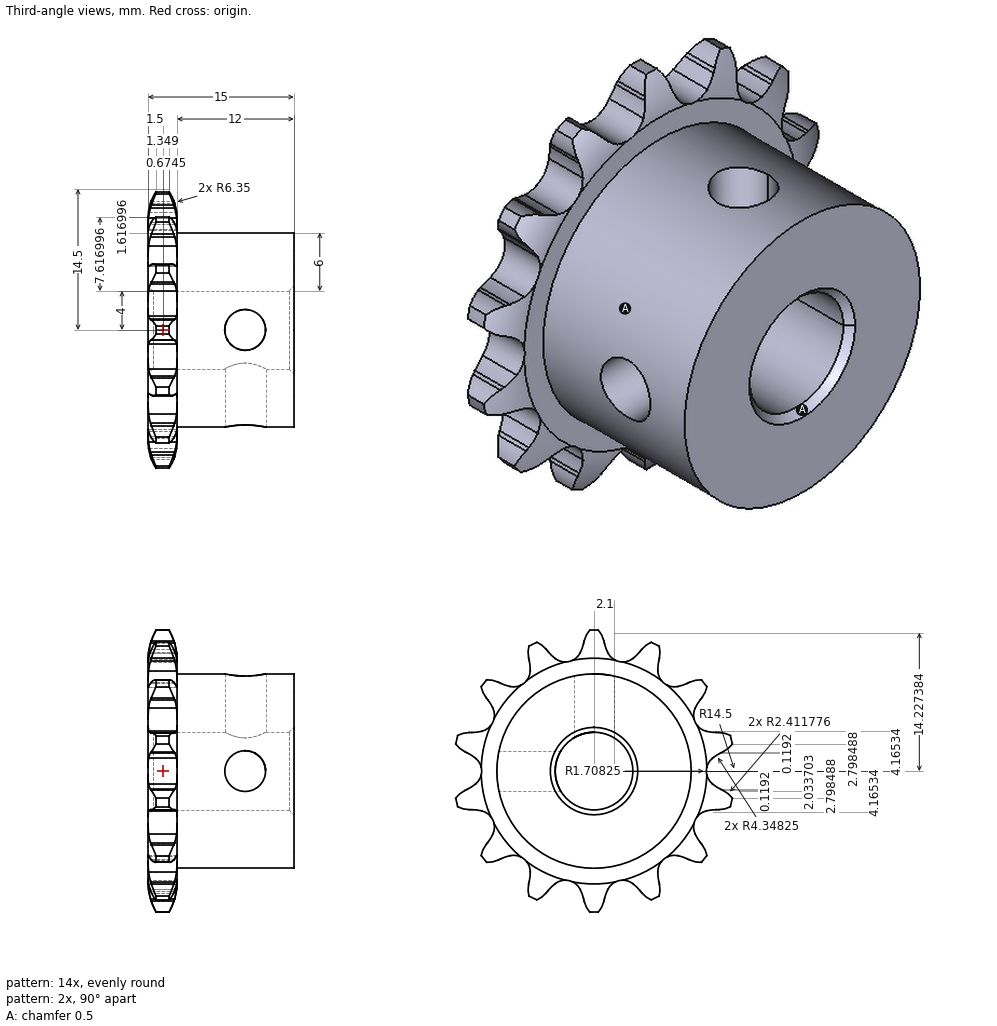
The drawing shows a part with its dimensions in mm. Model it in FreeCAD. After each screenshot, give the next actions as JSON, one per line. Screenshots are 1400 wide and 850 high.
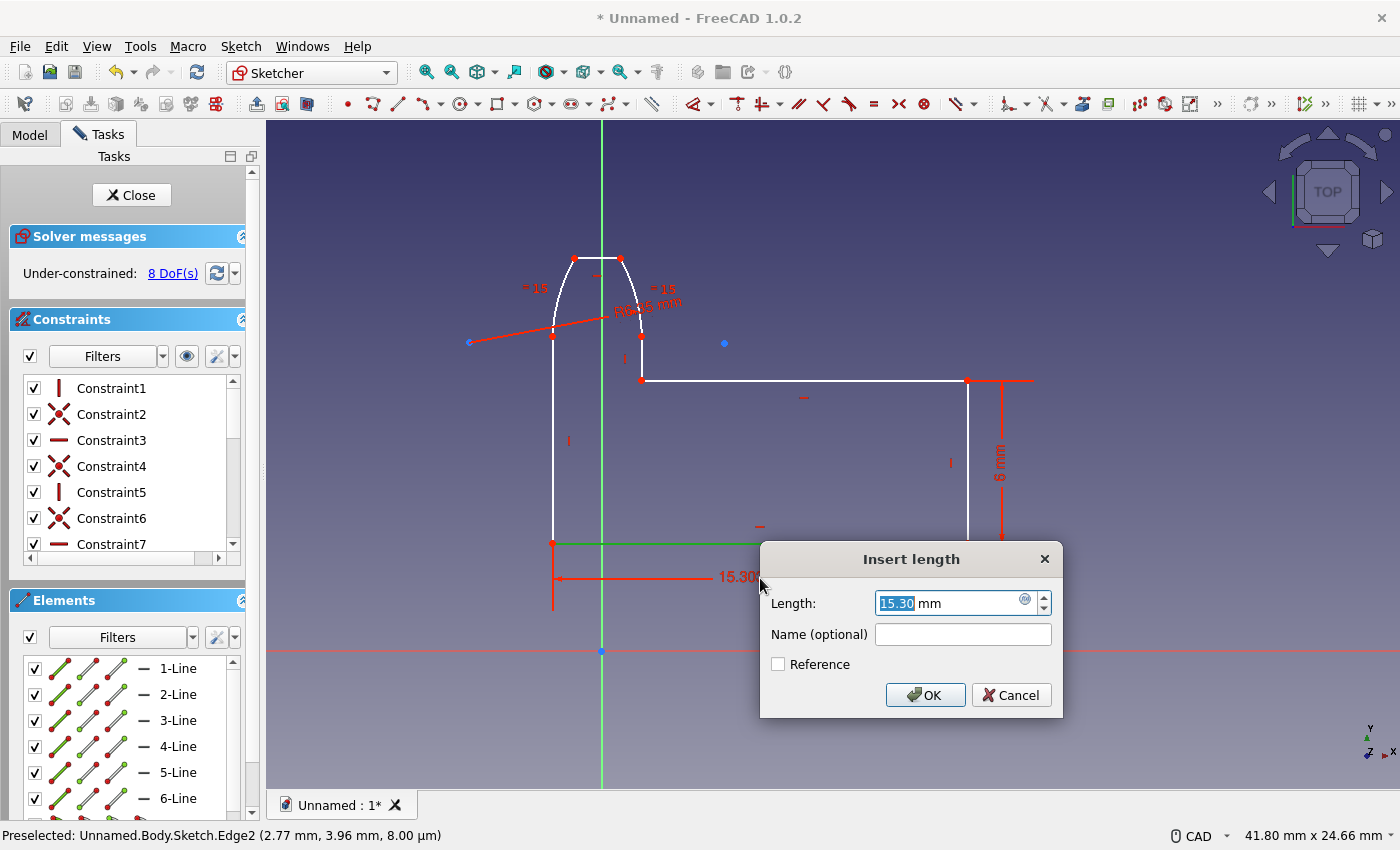
{"action": "type", "text": "15"}
{"action": "key", "text": "Return"}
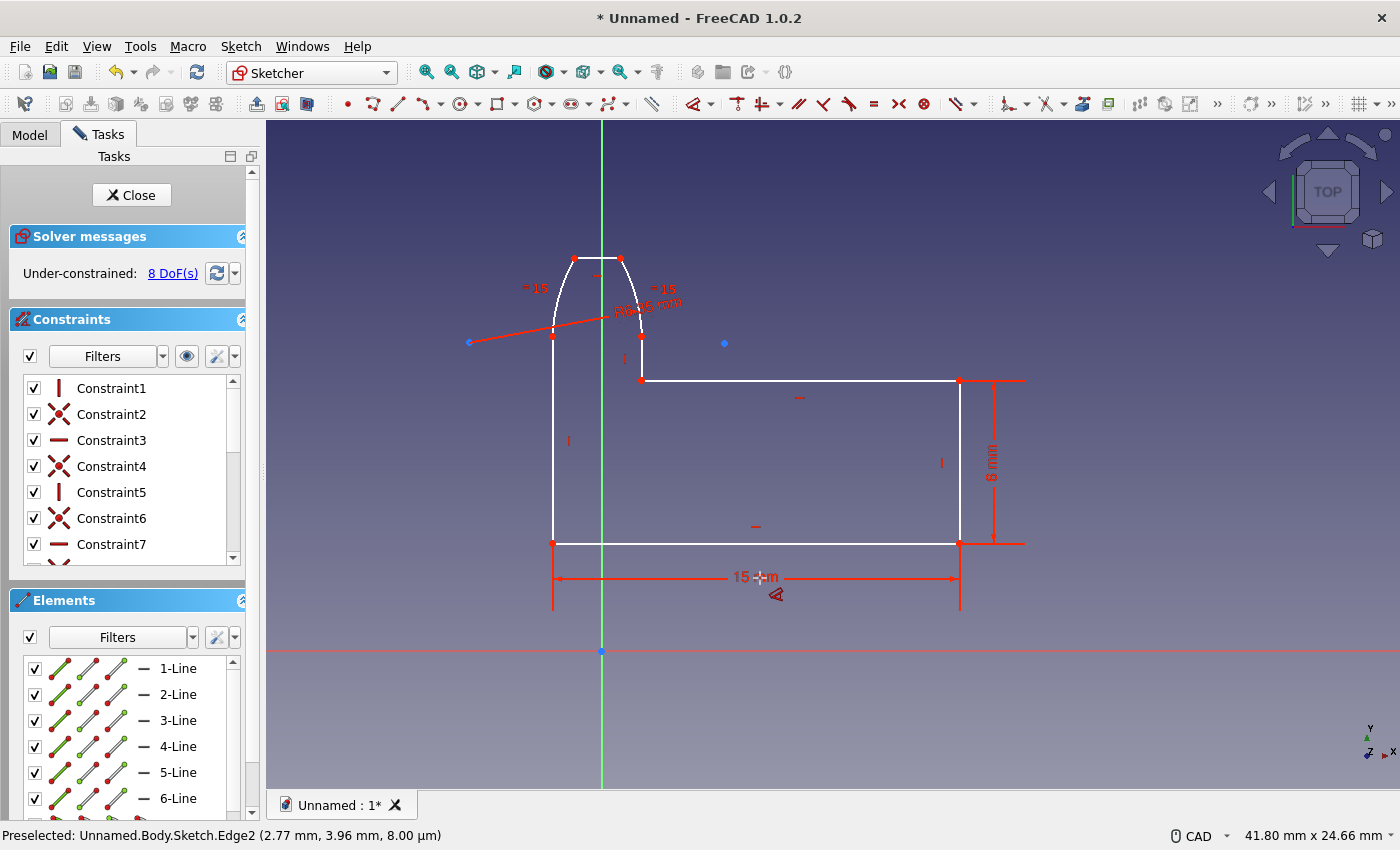
{"action": "left_click", "coordinate": [864, 381]}
{"action": "left_click", "coordinate": [801, 347]}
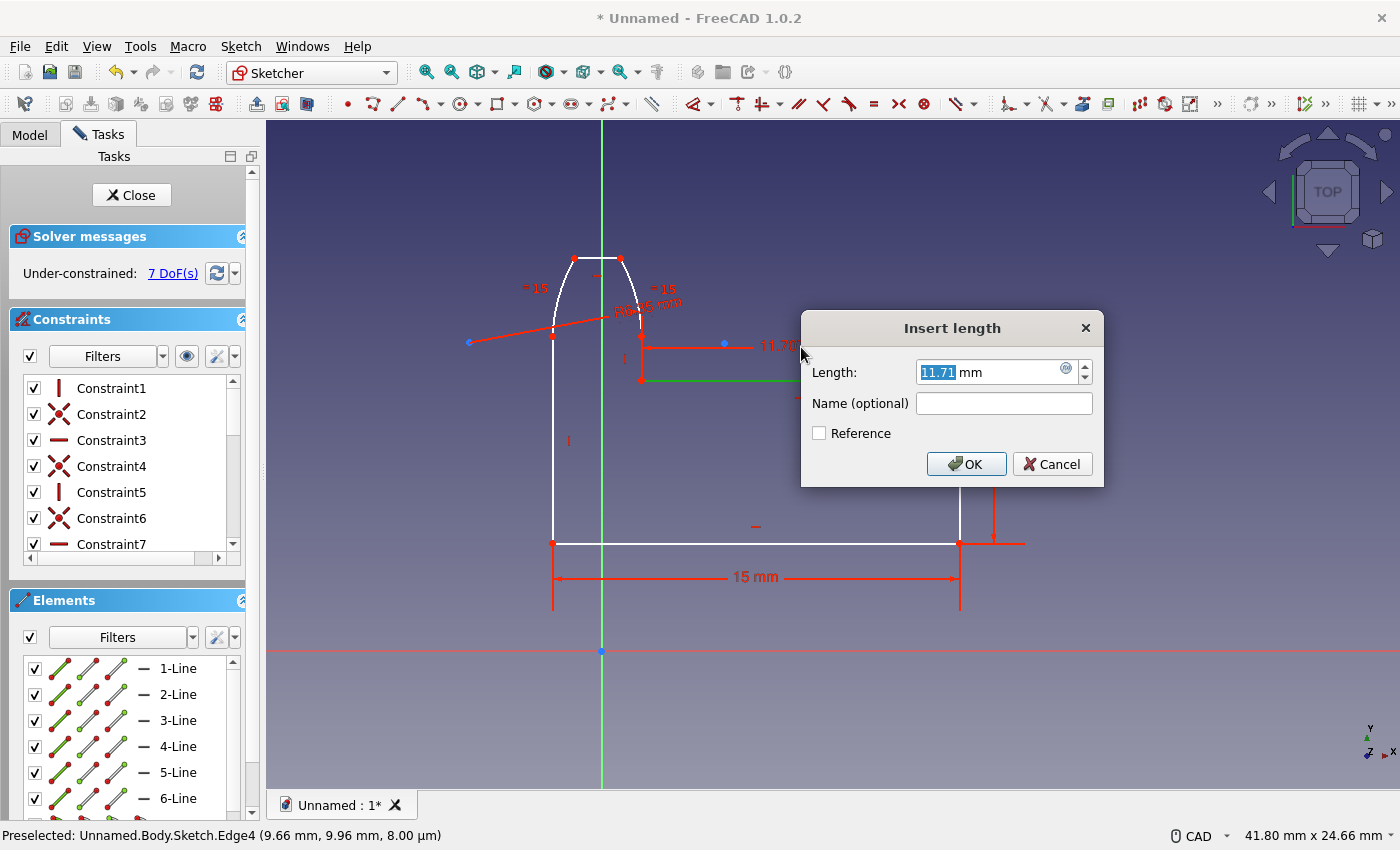
{"action": "type", "text": "12"}
{"action": "key", "text": "Return"}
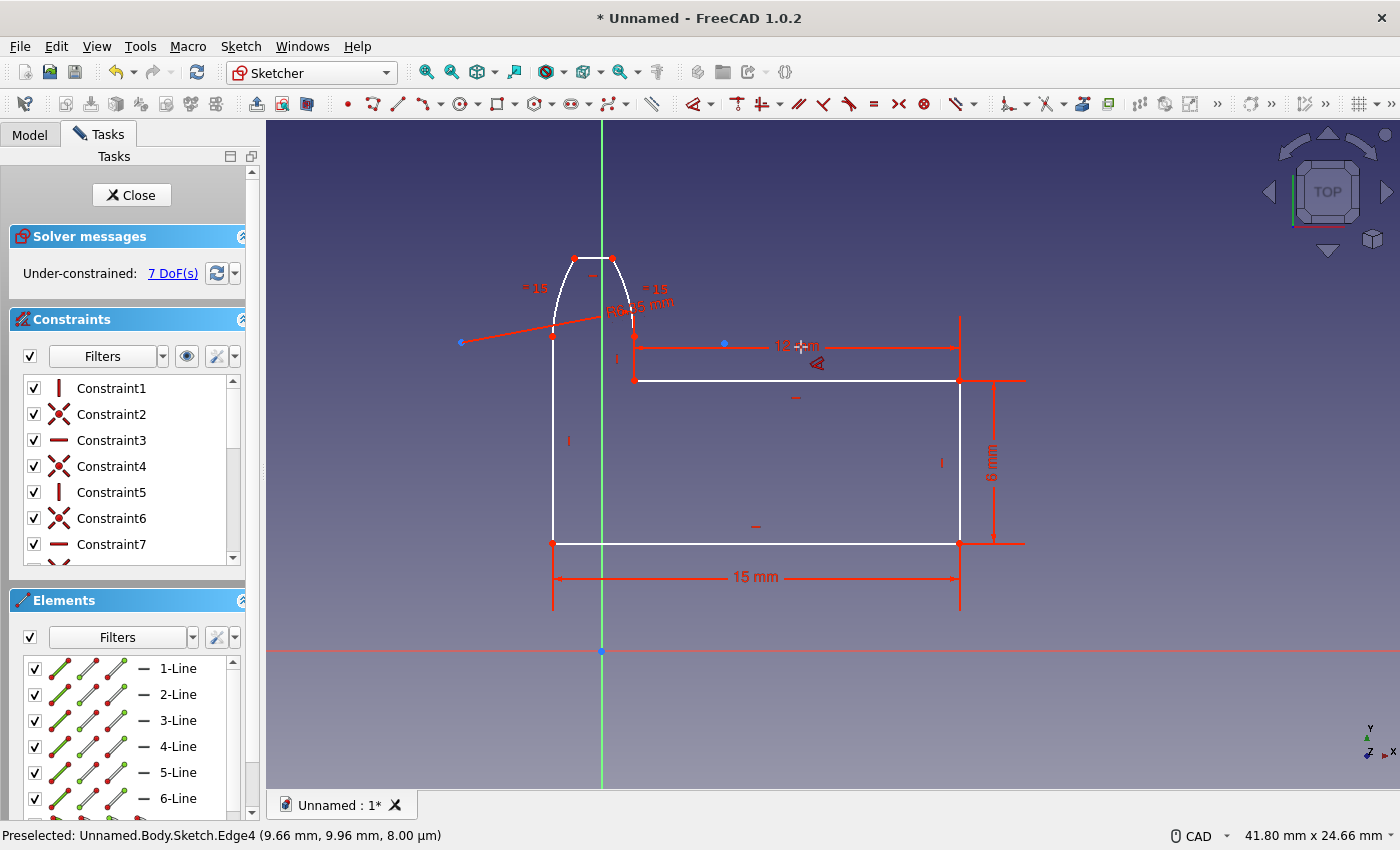
{"action": "left_click", "coordinate": [553, 544]}
{"action": "left_click", "coordinate": [519, 597]}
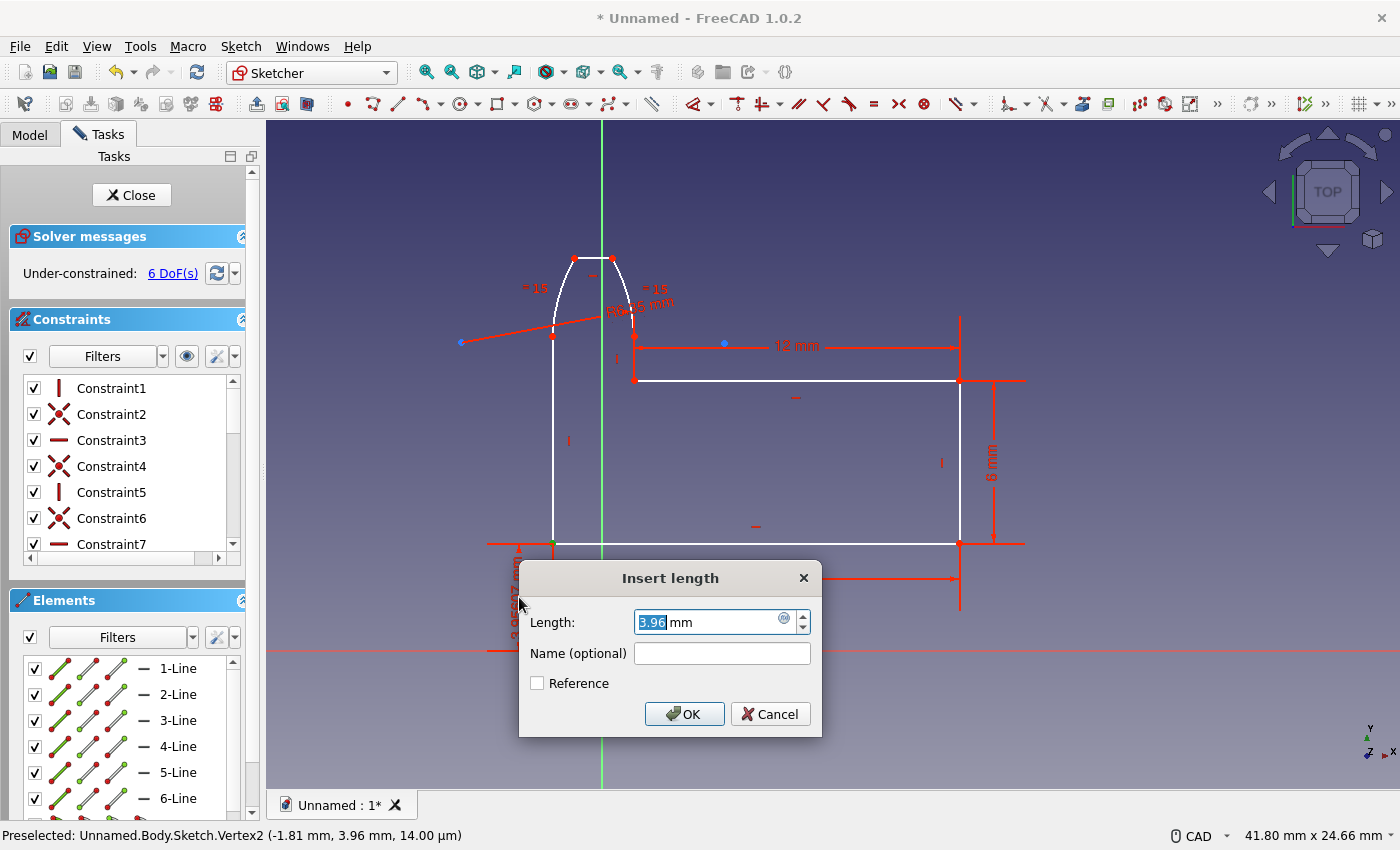
{"action": "type", "text": "4"}
{"action": "key", "text": "Return"}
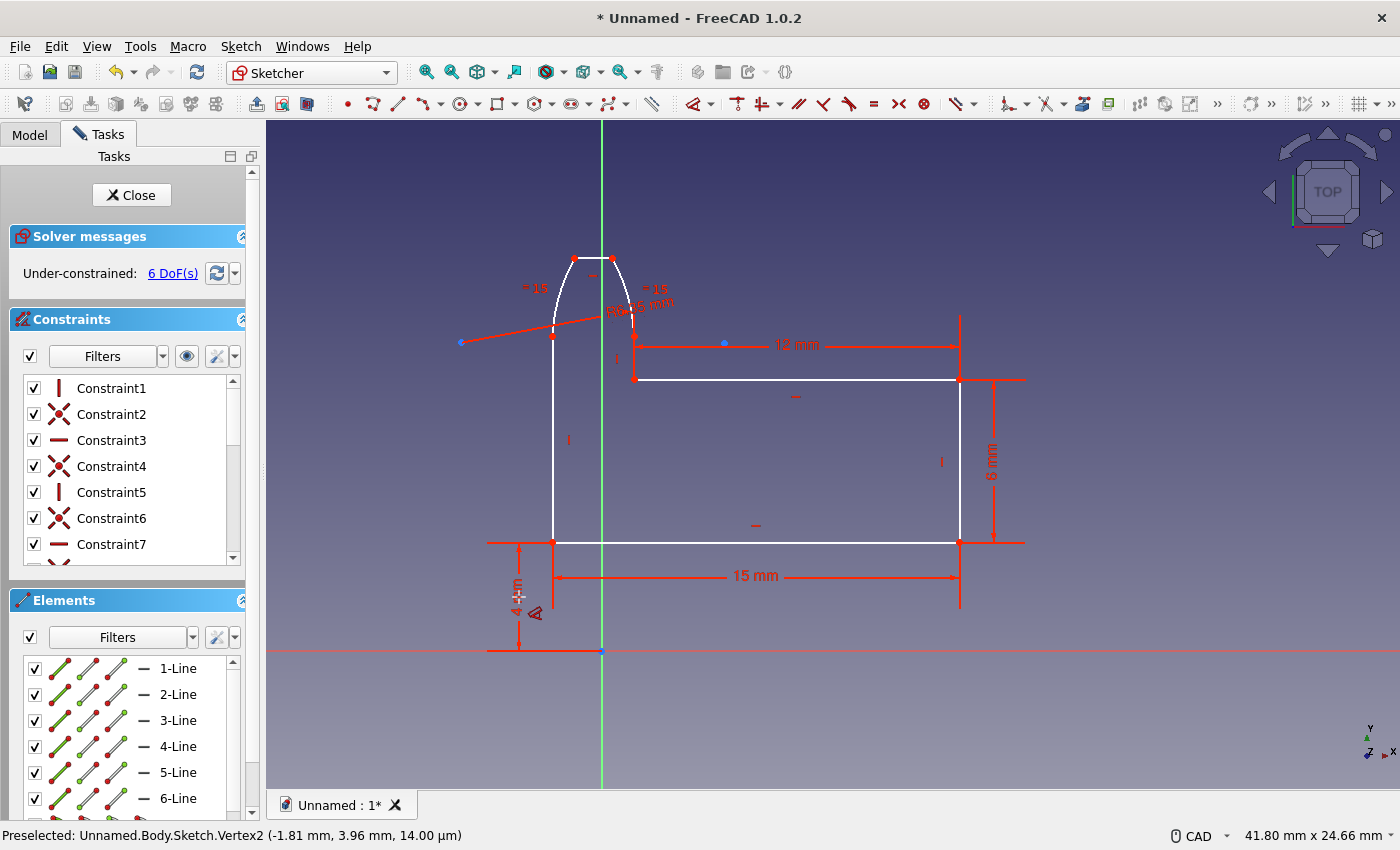
{"action": "left_click", "coordinate": [553, 337]}
{"action": "left_click", "coordinate": [577, 685]}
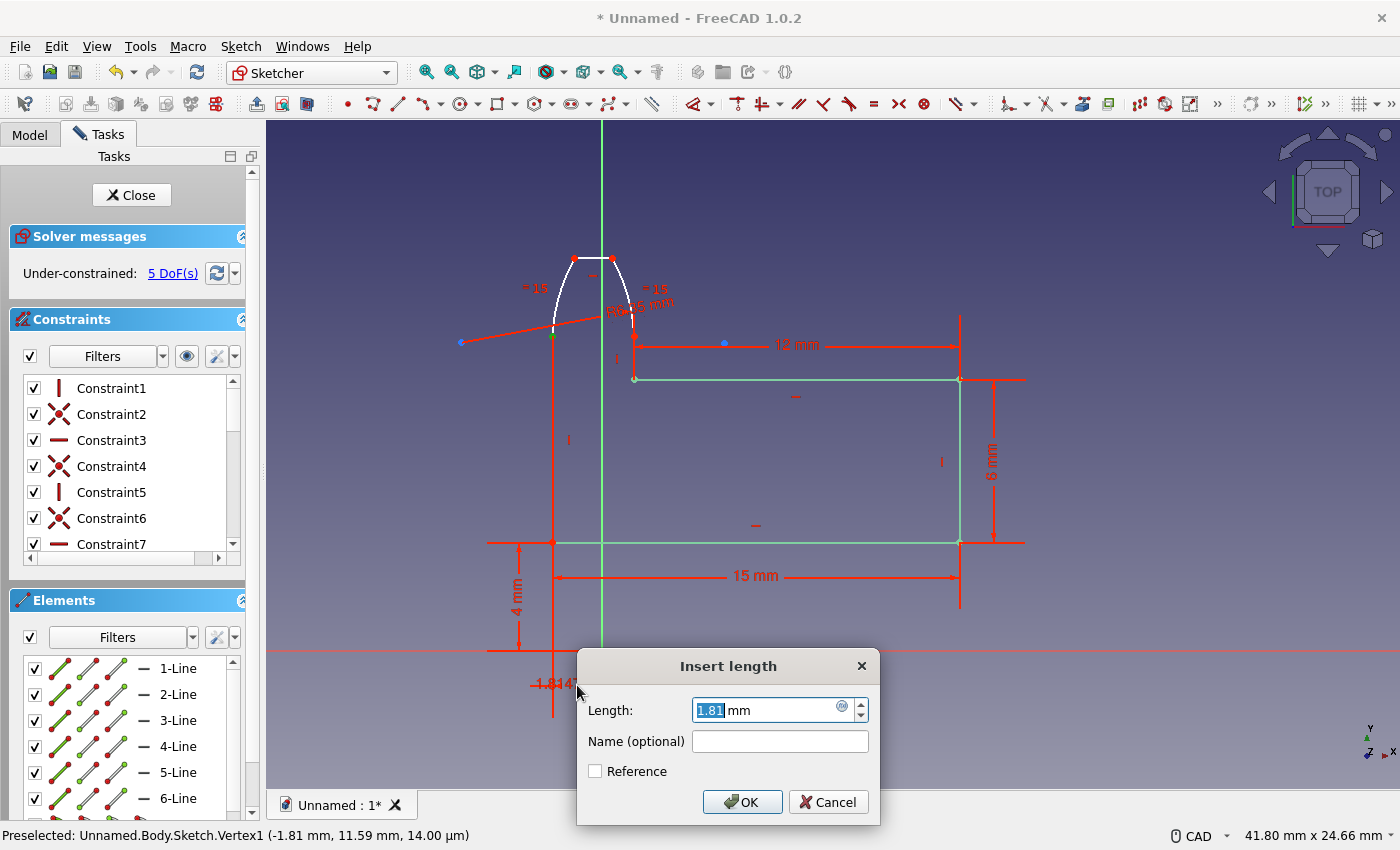
{"action": "type", "text": "1.5"}
{"action": "key", "text": "Return"}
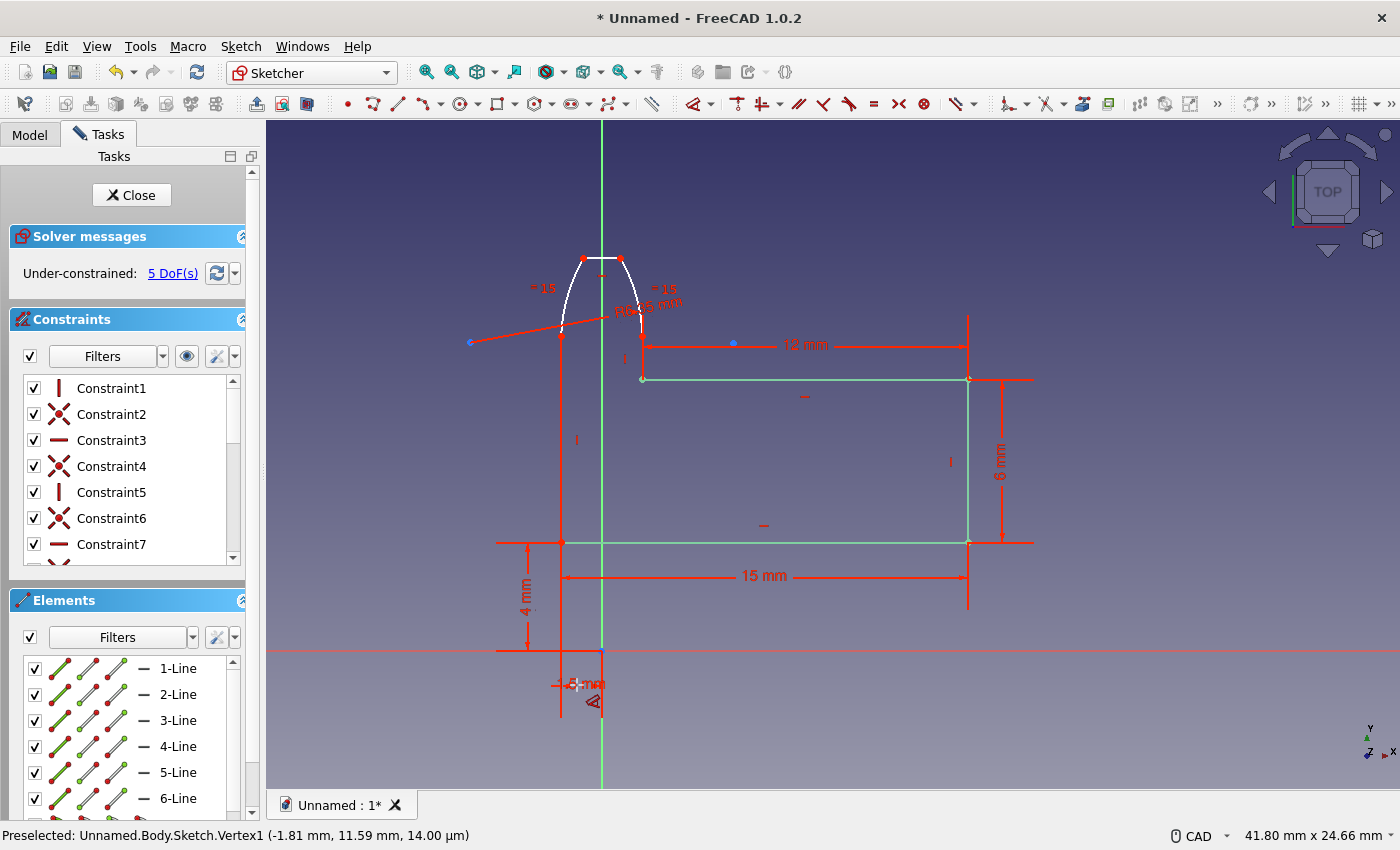
{"action": "left_click", "coordinate": [606, 258]}
{"action": "left_click", "coordinate": [615, 224]}